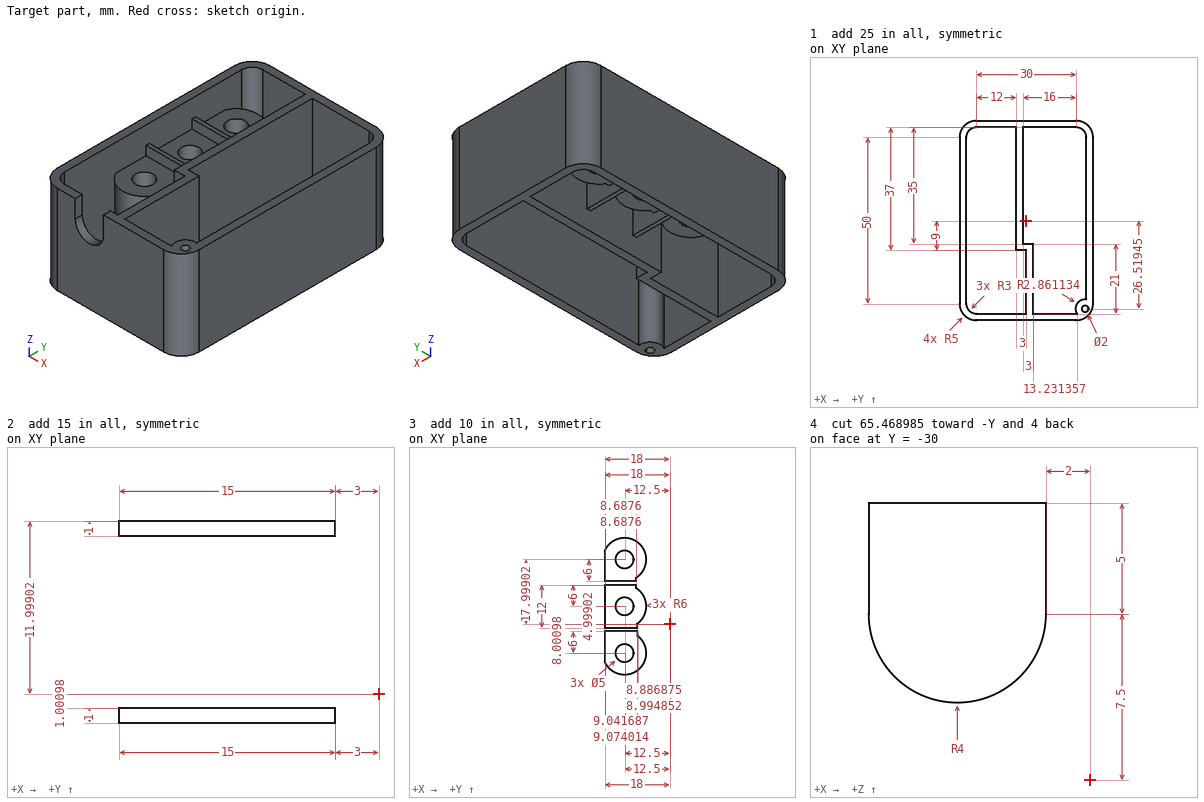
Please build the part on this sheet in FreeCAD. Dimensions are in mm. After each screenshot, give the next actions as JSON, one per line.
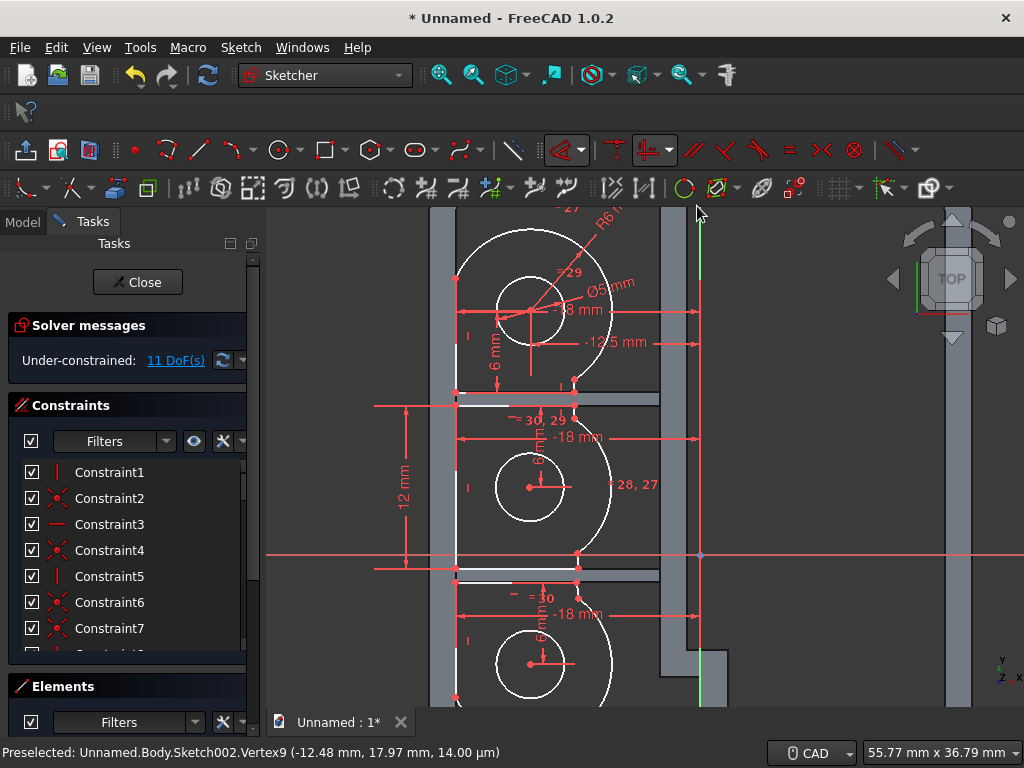
{"action": "left_click", "coordinate": [530, 487]}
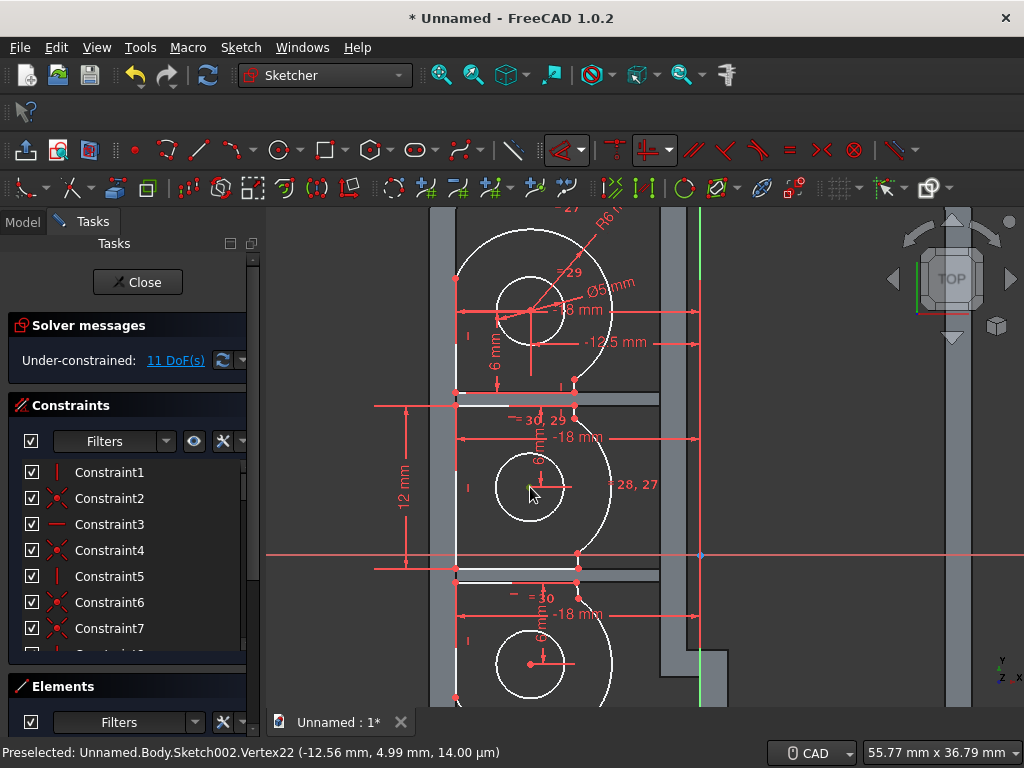
{"action": "left_click", "coordinate": [584, 150]}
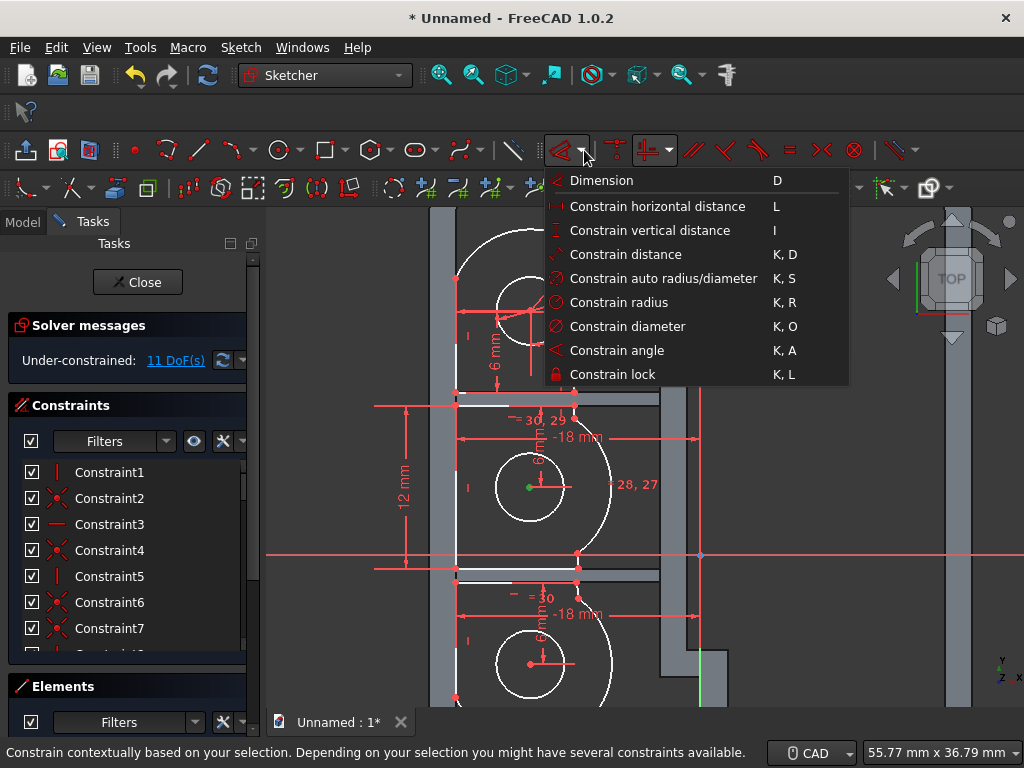
{"action": "left_click", "coordinate": [697, 206]}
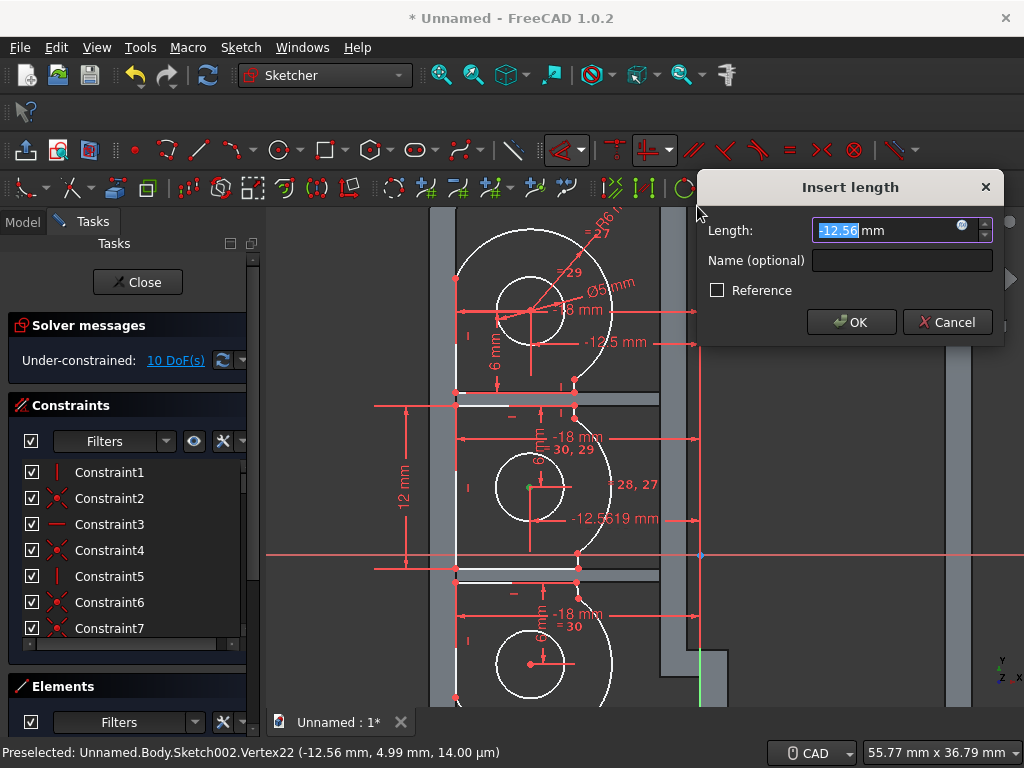
{"action": "type", "text": "-12.5"}
{"action": "key", "text": "Return"}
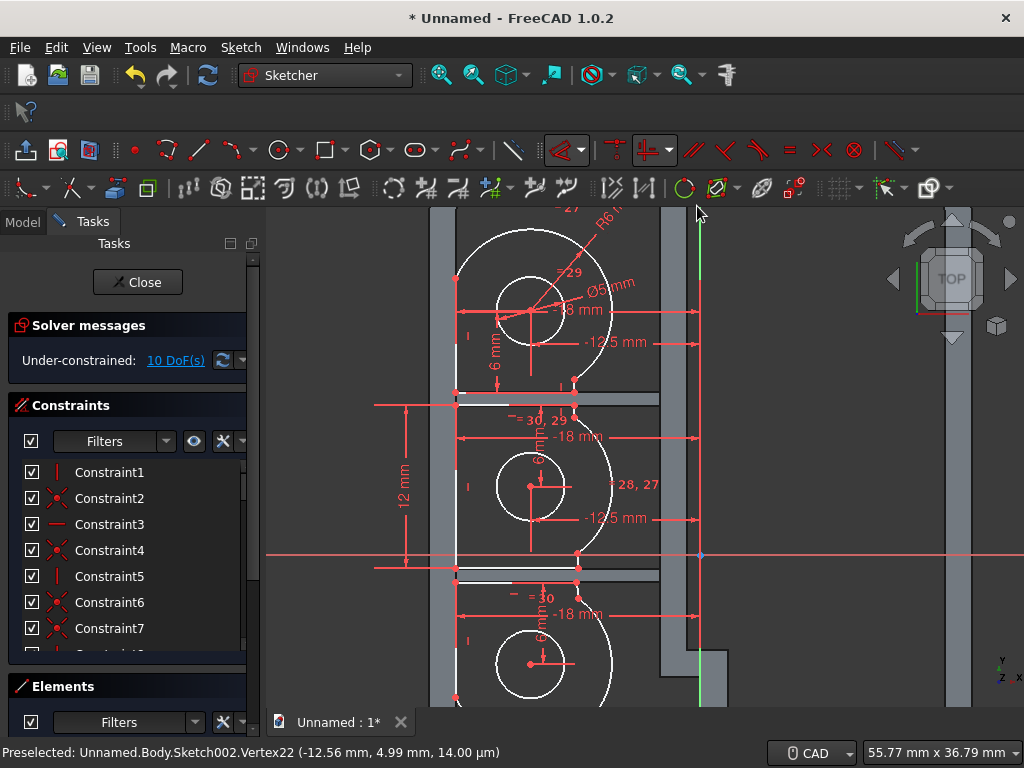
{"action": "left_click", "coordinate": [530, 664]}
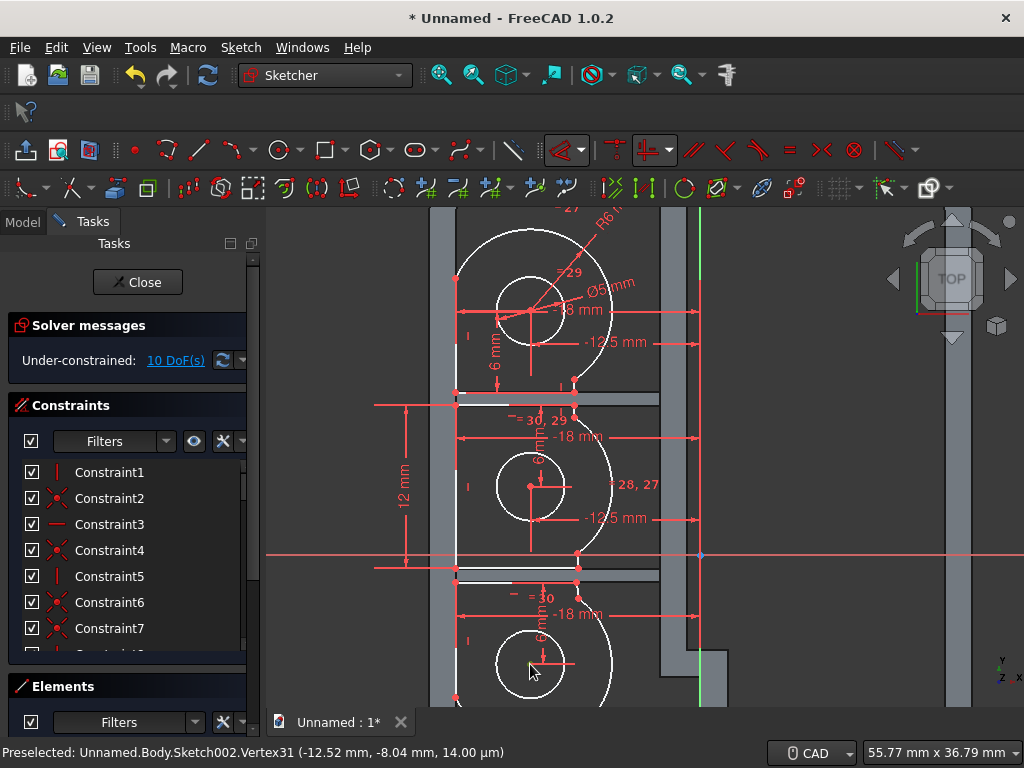
{"action": "key", "text": "l"}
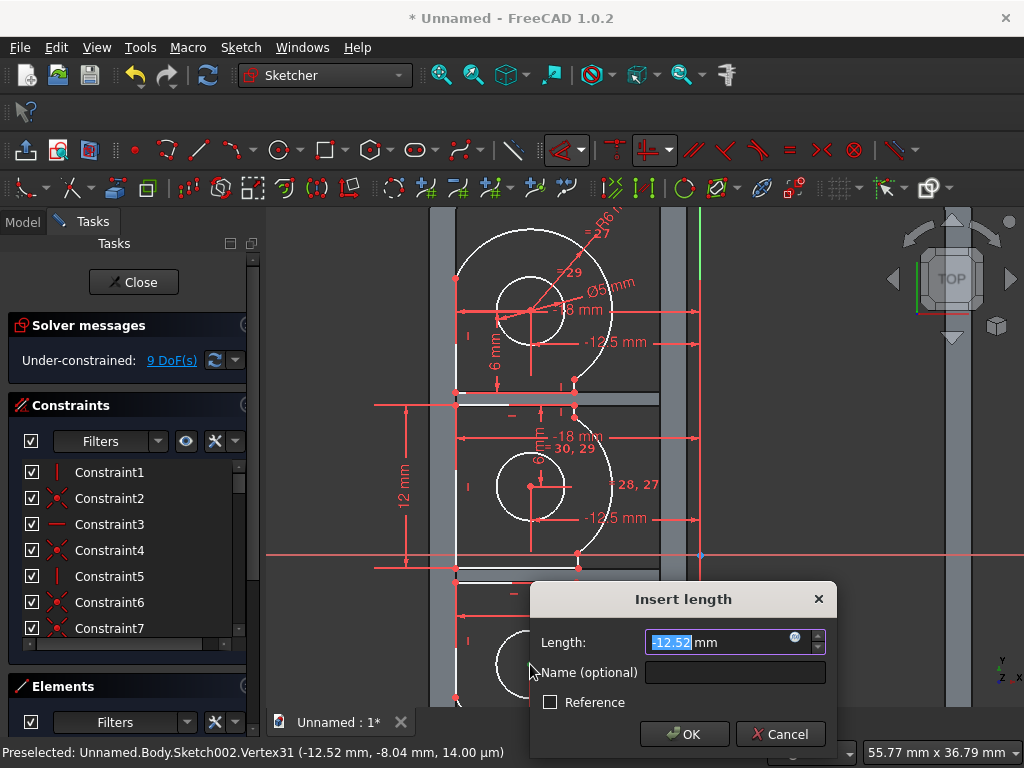
{"action": "type", "text": "-12.5"}
{"action": "key", "text": "Return"}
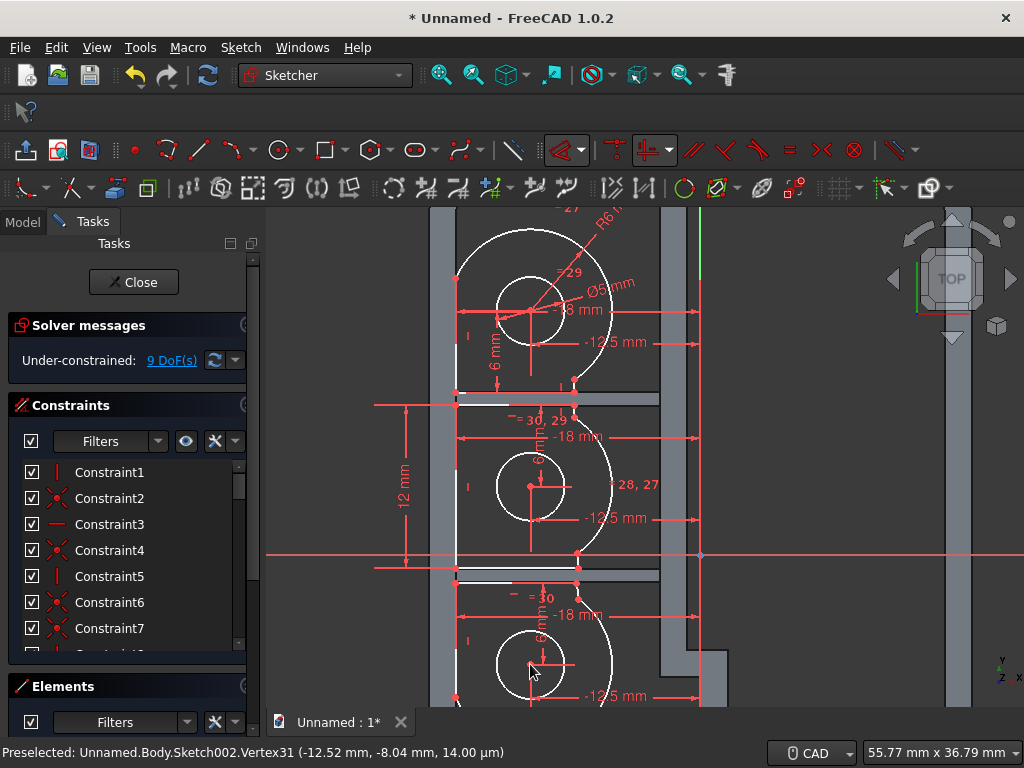
{"action": "left_click", "coordinate": [491, 393]}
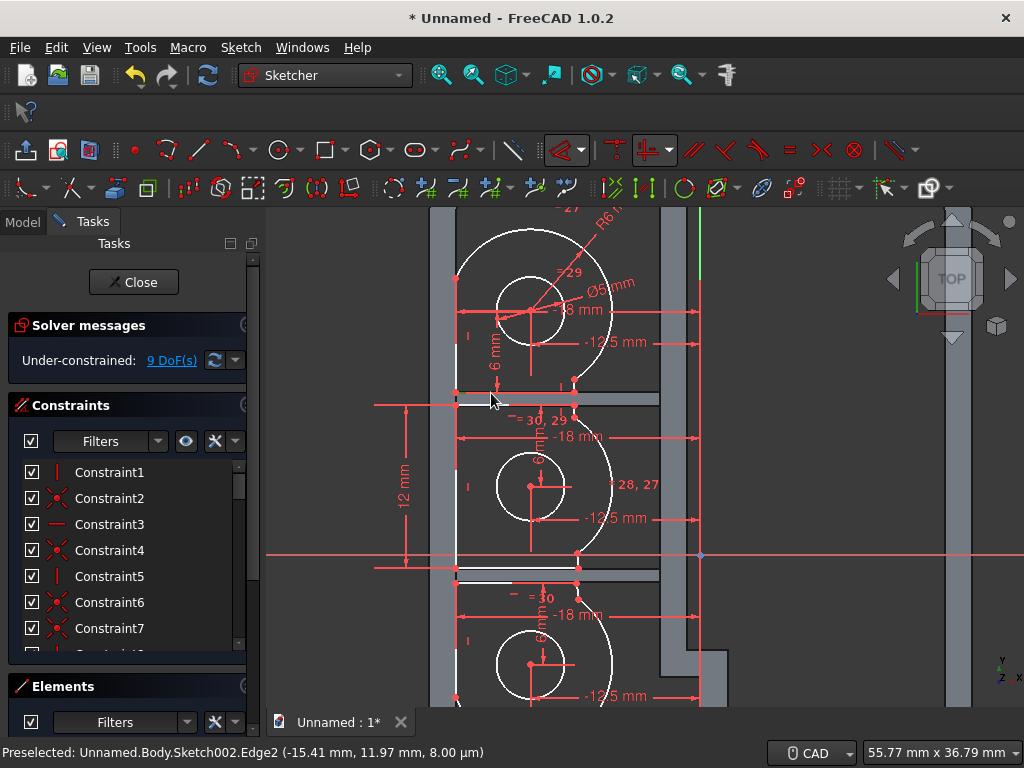
{"action": "left_click", "coordinate": [584, 150]}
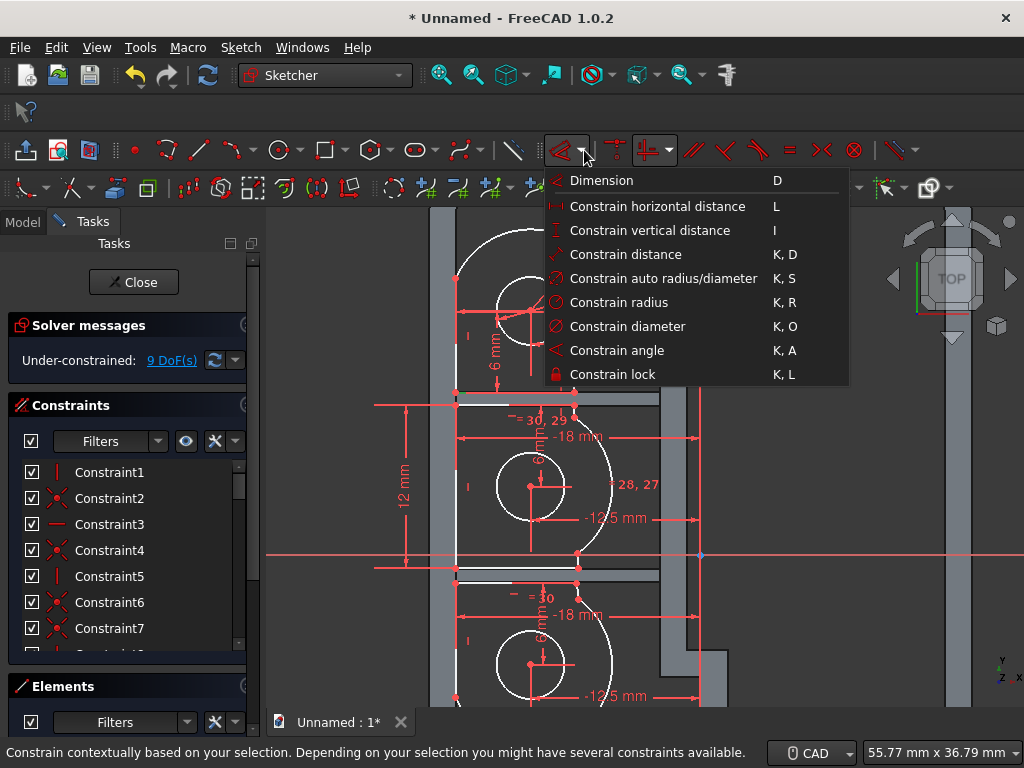
{"action": "left_click", "coordinate": [697, 206]}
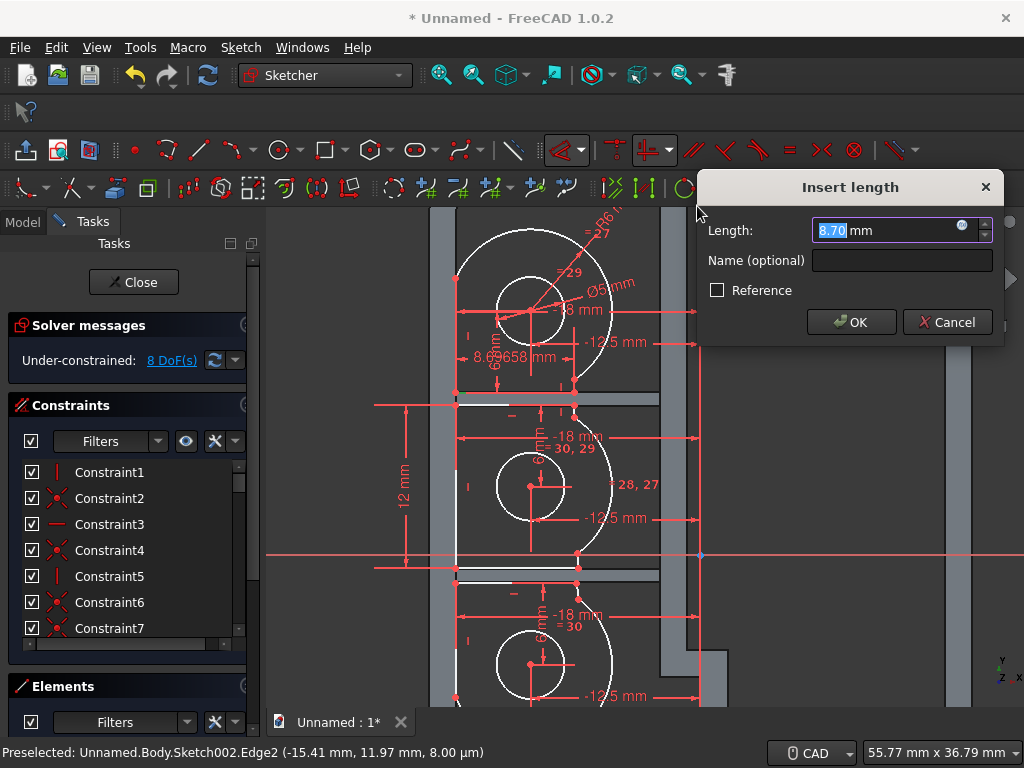
{"action": "type", "text": "8.6876"}
{"action": "key", "text": "Return"}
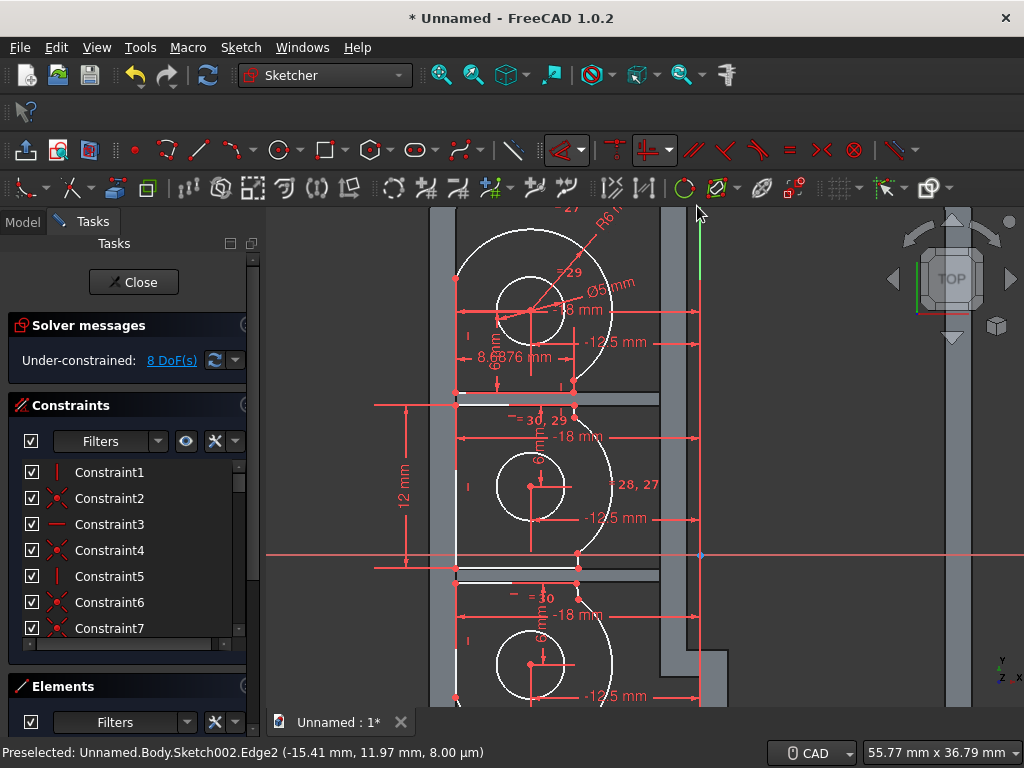
{"action": "left_click", "coordinate": [539, 405]}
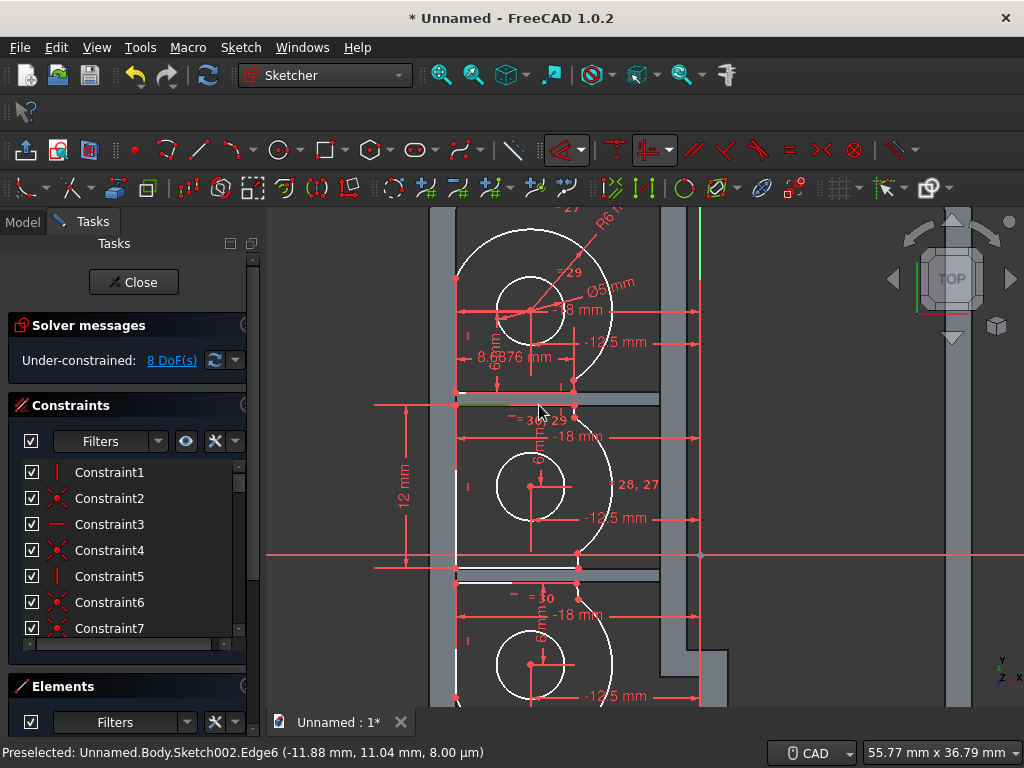
{"action": "left_click", "coordinate": [584, 150]}